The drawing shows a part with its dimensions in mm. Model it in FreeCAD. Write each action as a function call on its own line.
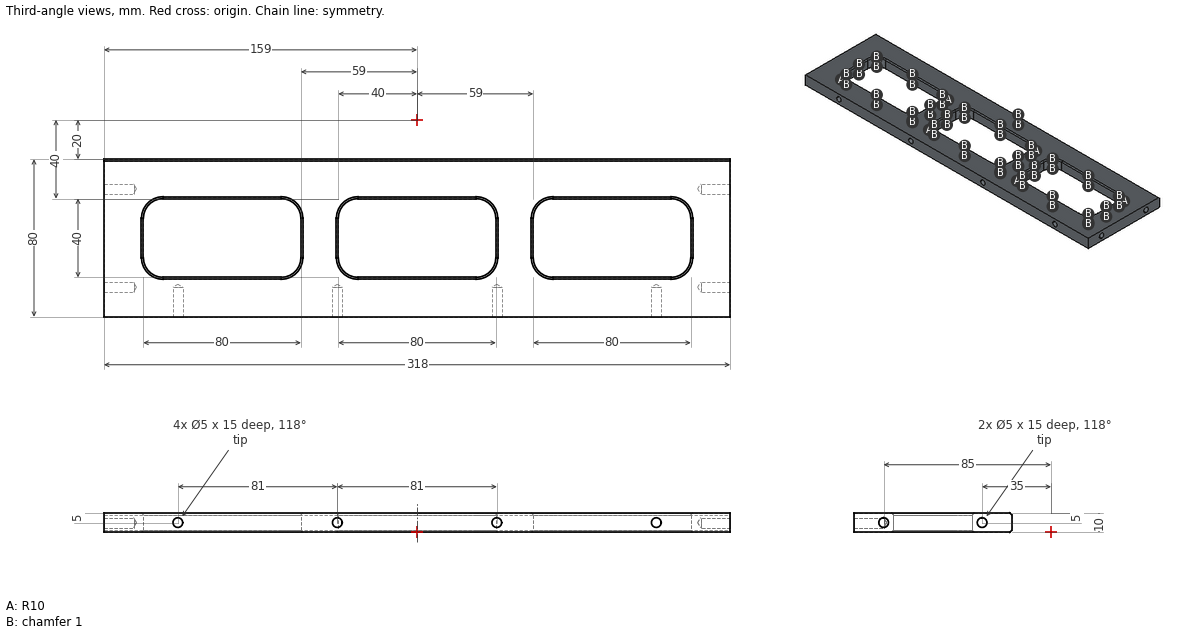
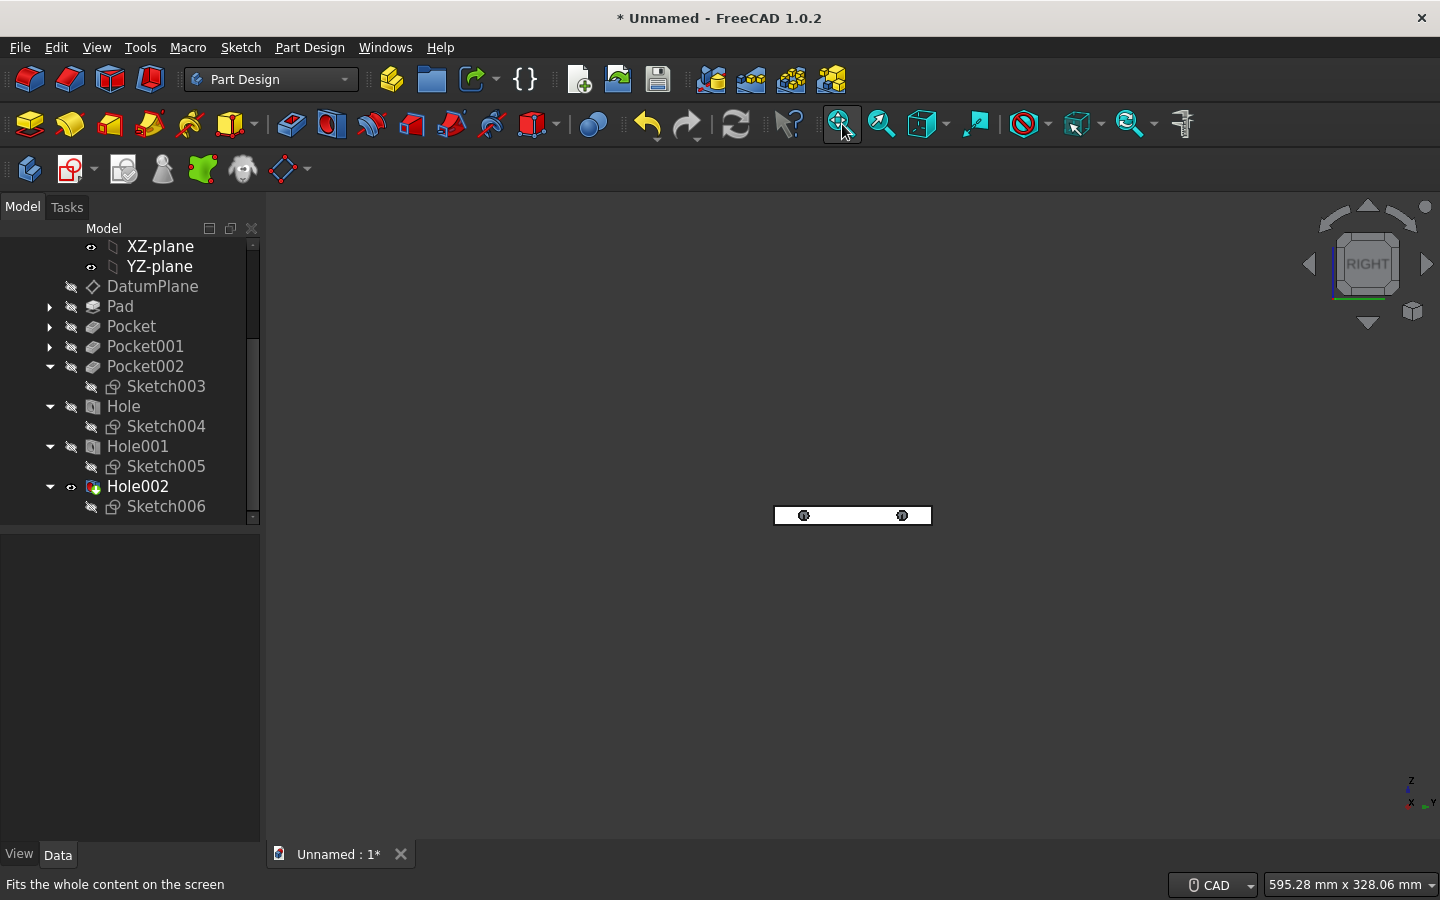
key(5)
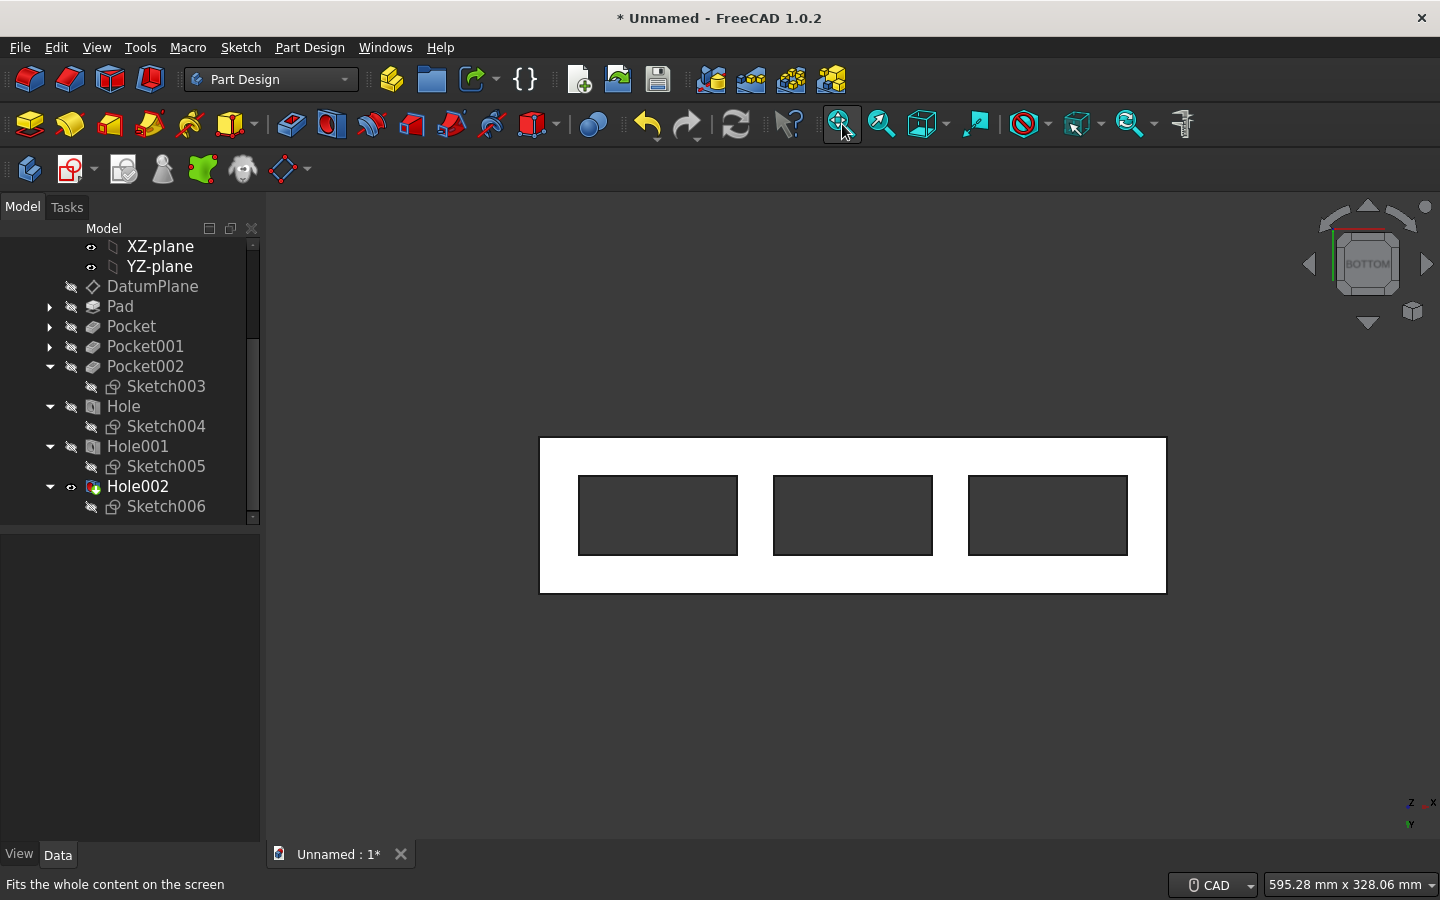
scroll(932, 475, up, 4)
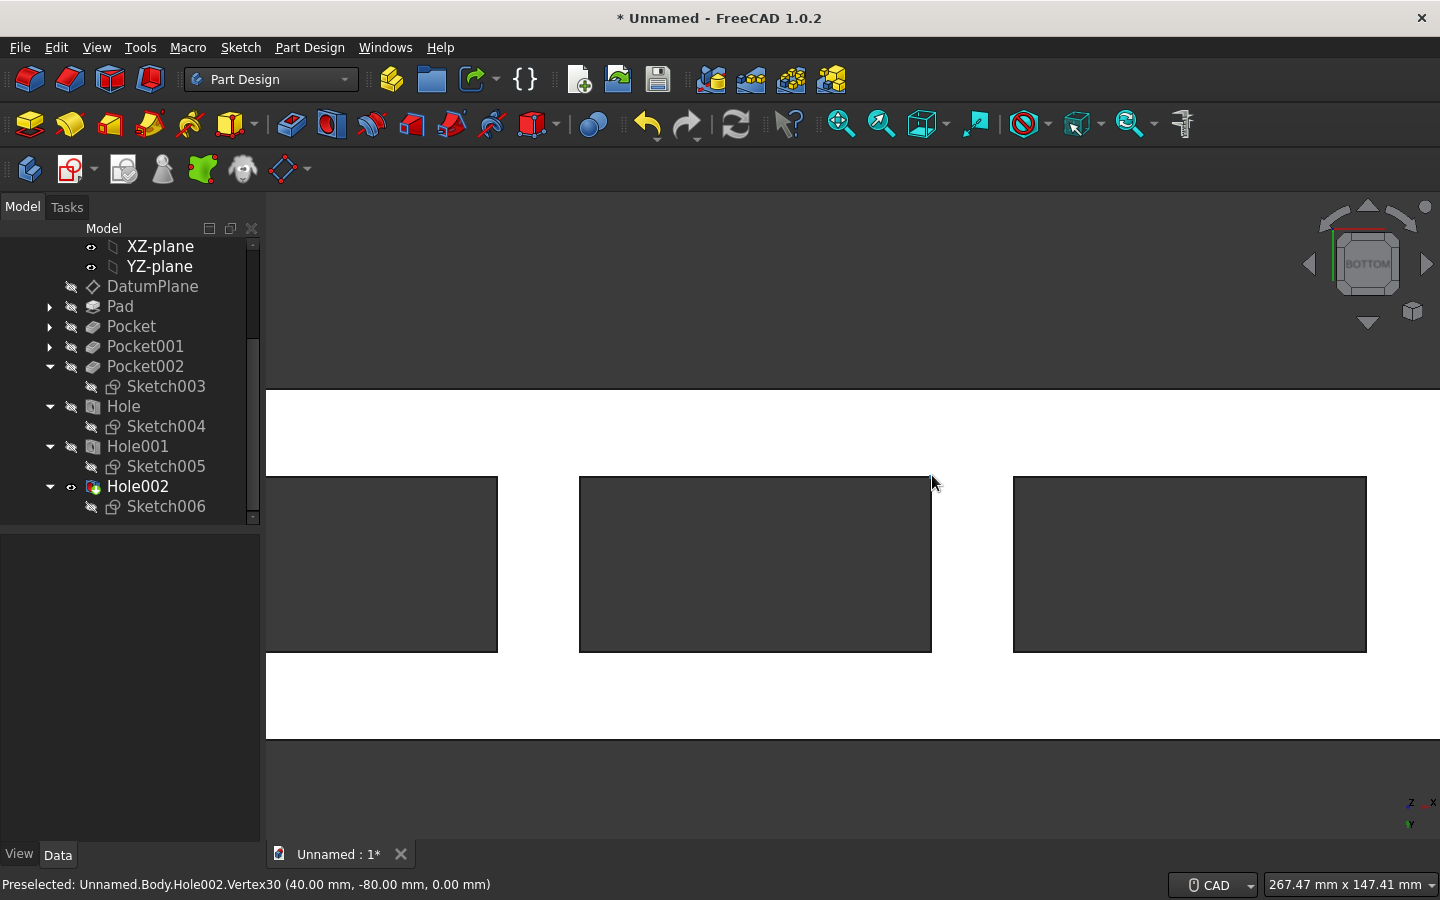
click(842, 124)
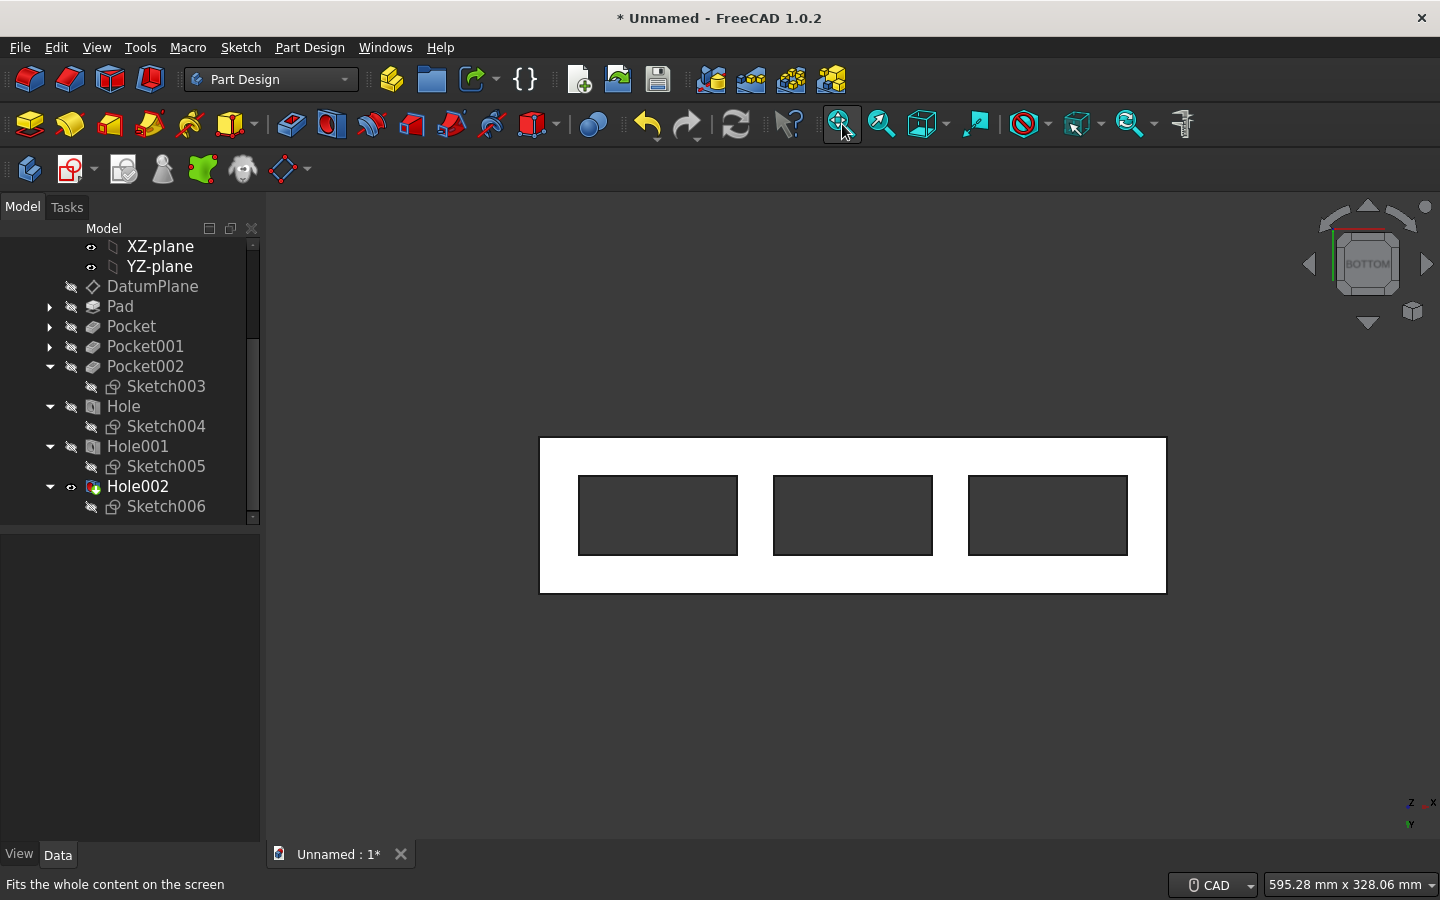
key(4)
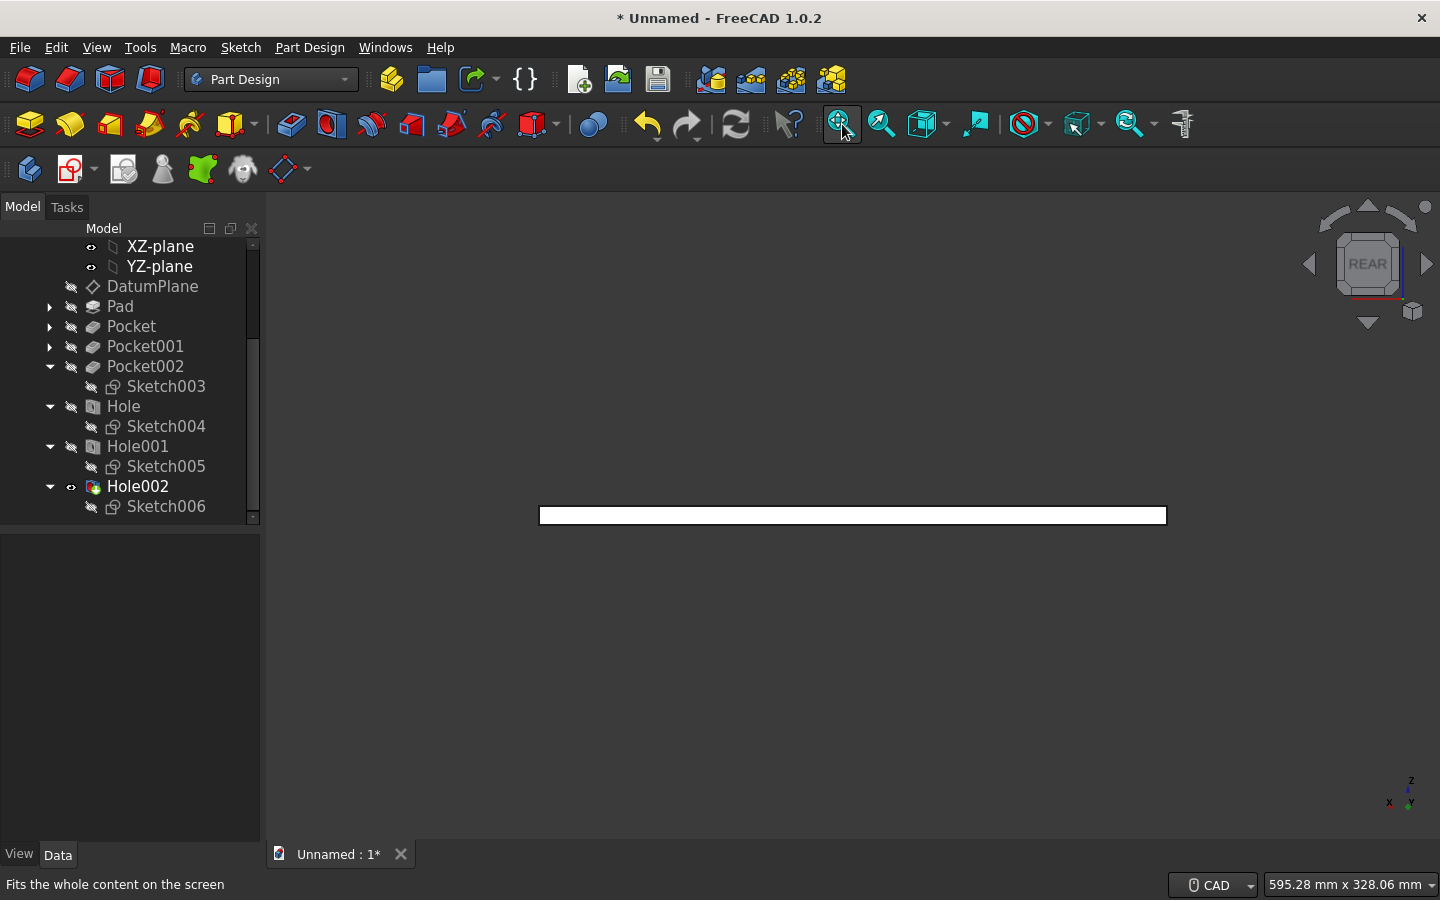
scroll(774, 514, up, 4)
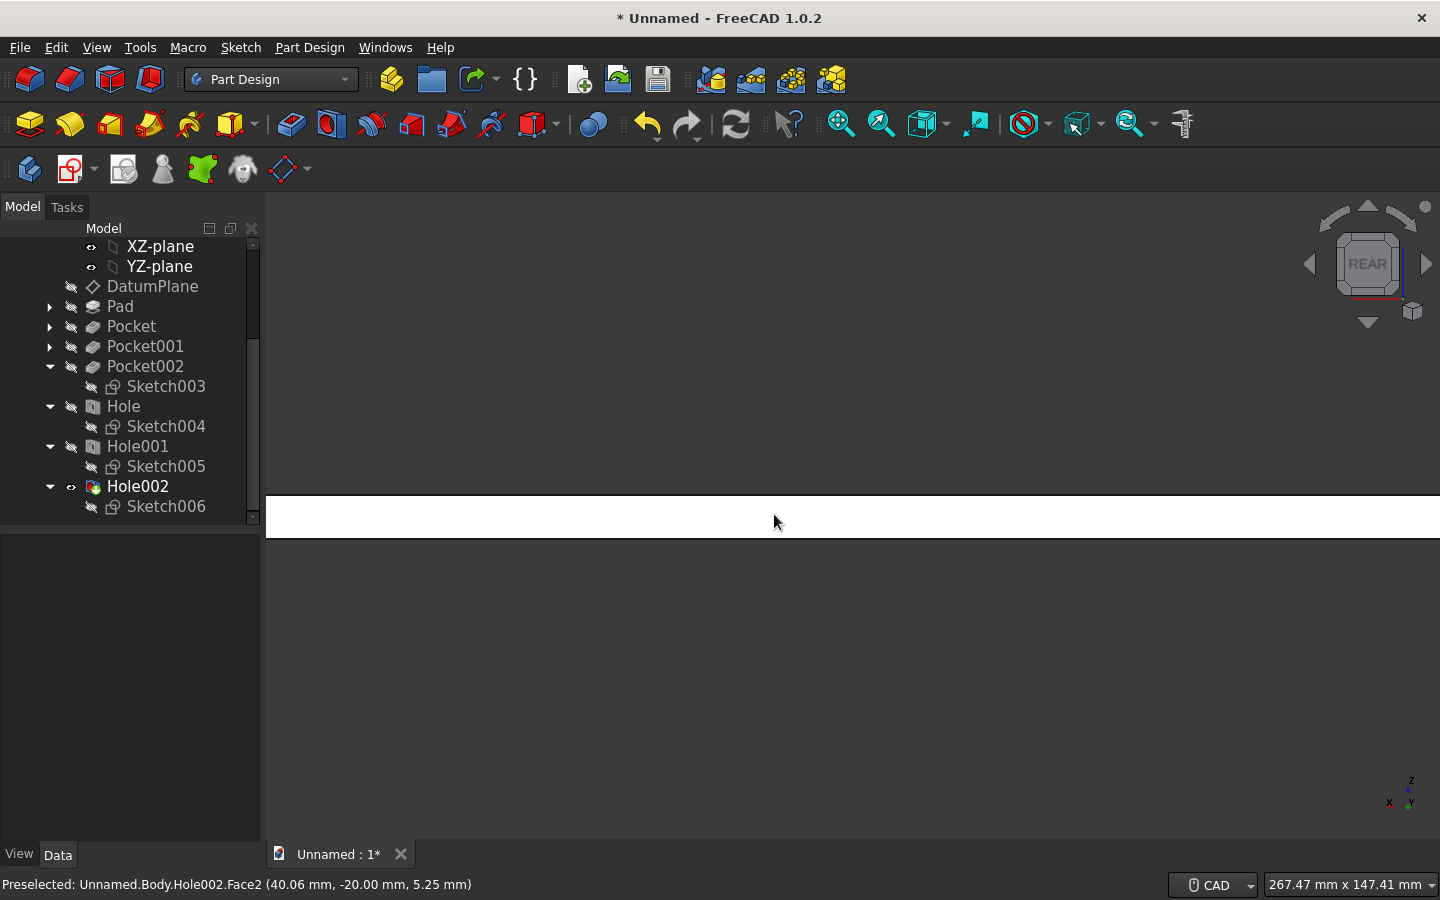
click(842, 124)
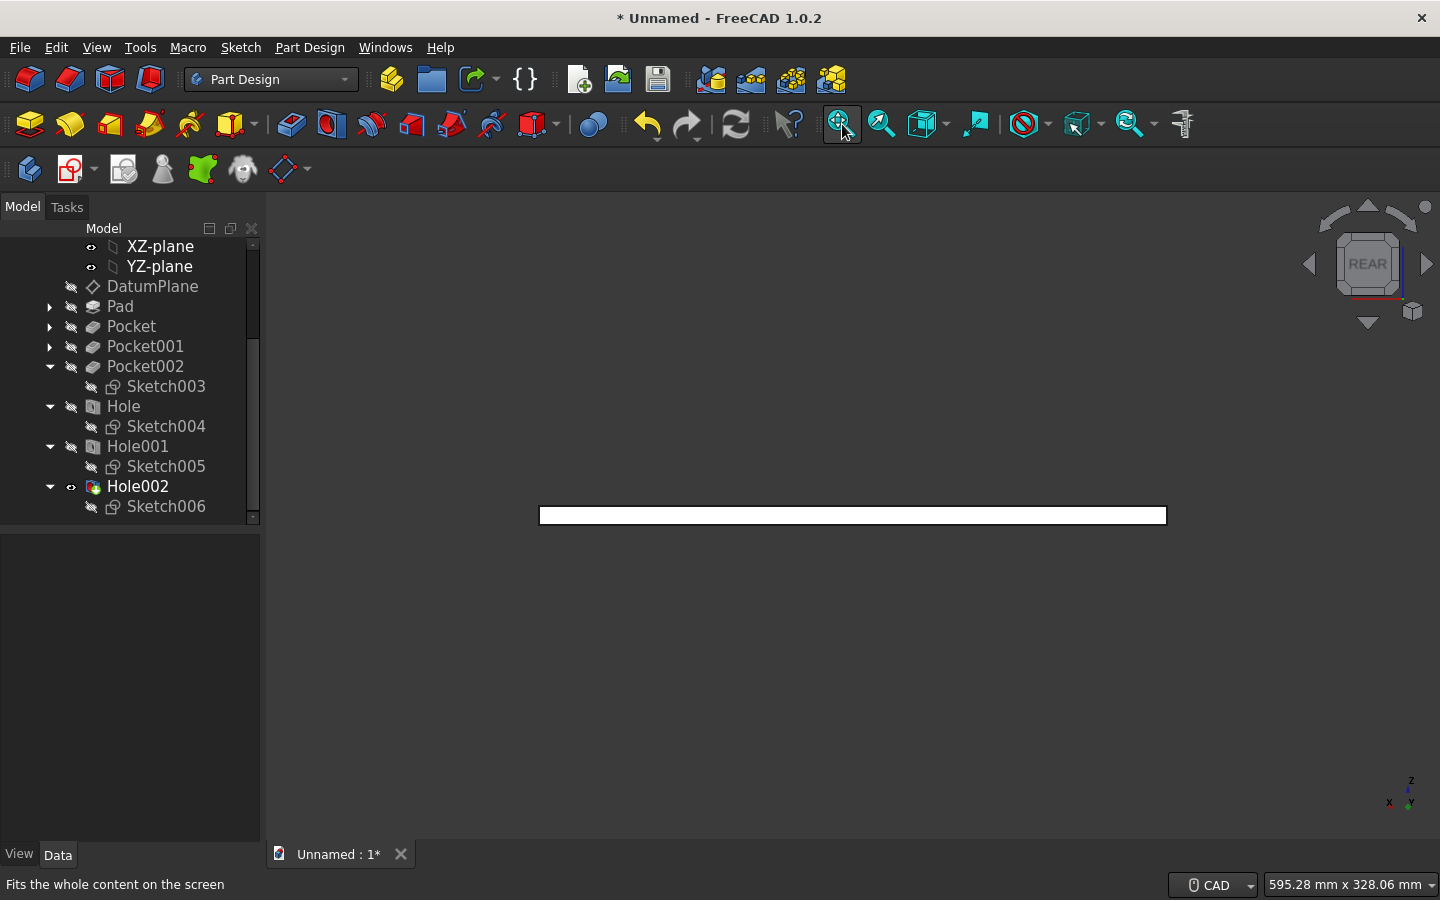
key(6)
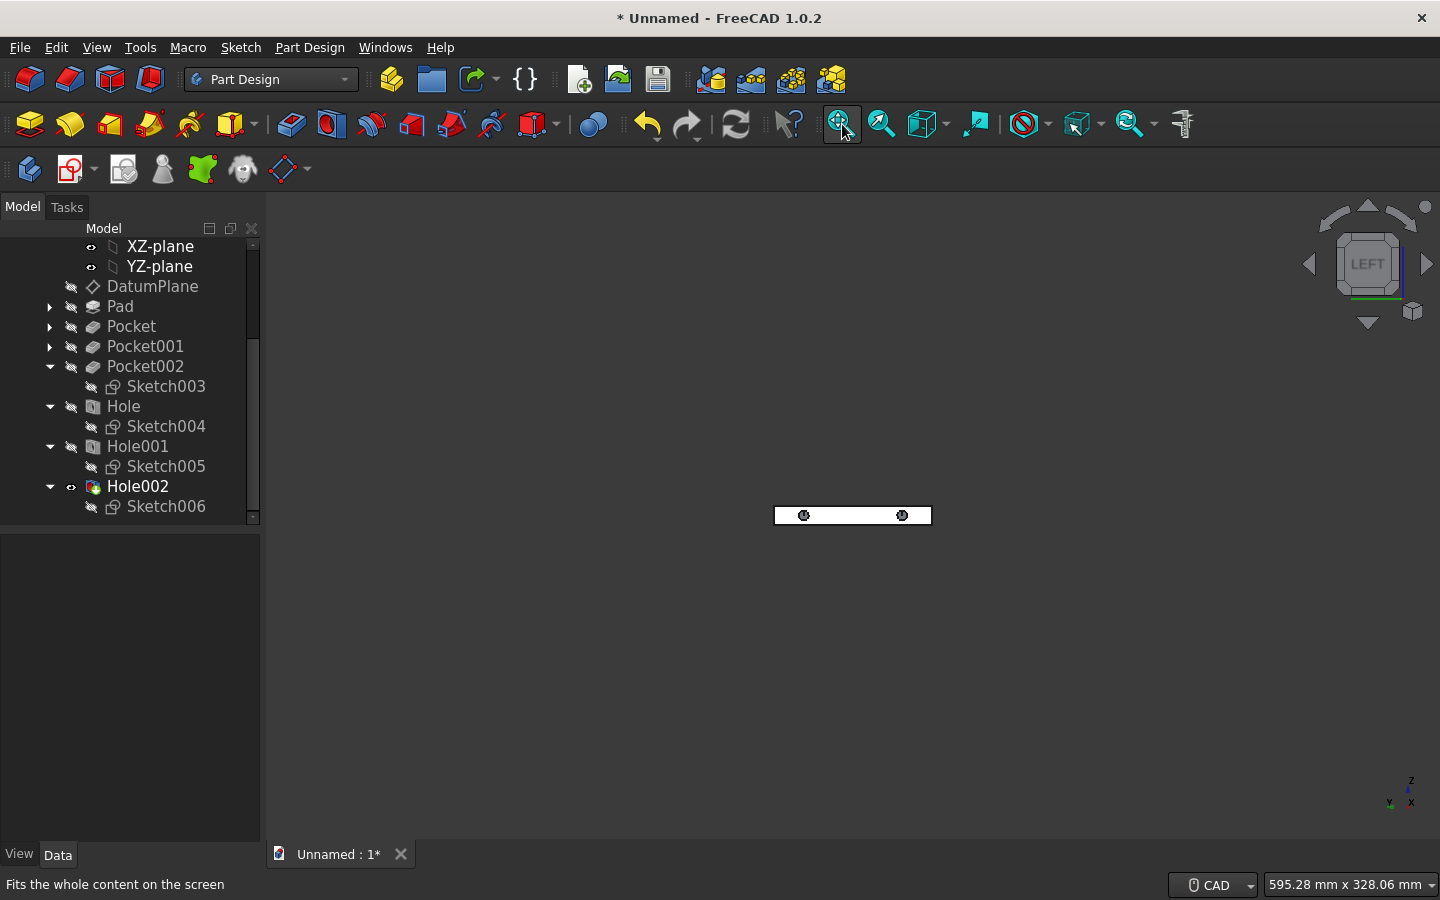
click(842, 124)